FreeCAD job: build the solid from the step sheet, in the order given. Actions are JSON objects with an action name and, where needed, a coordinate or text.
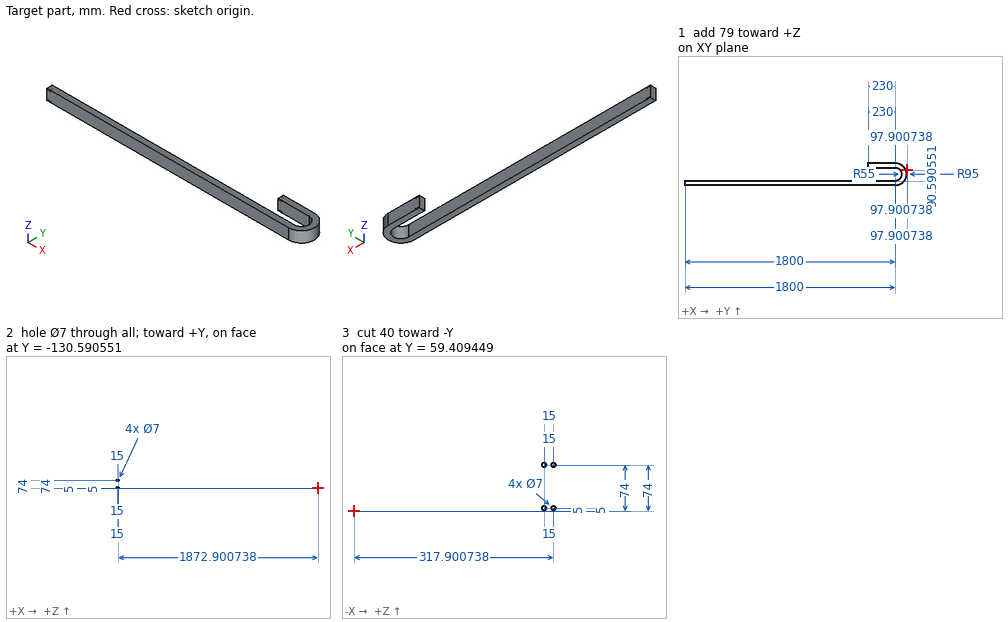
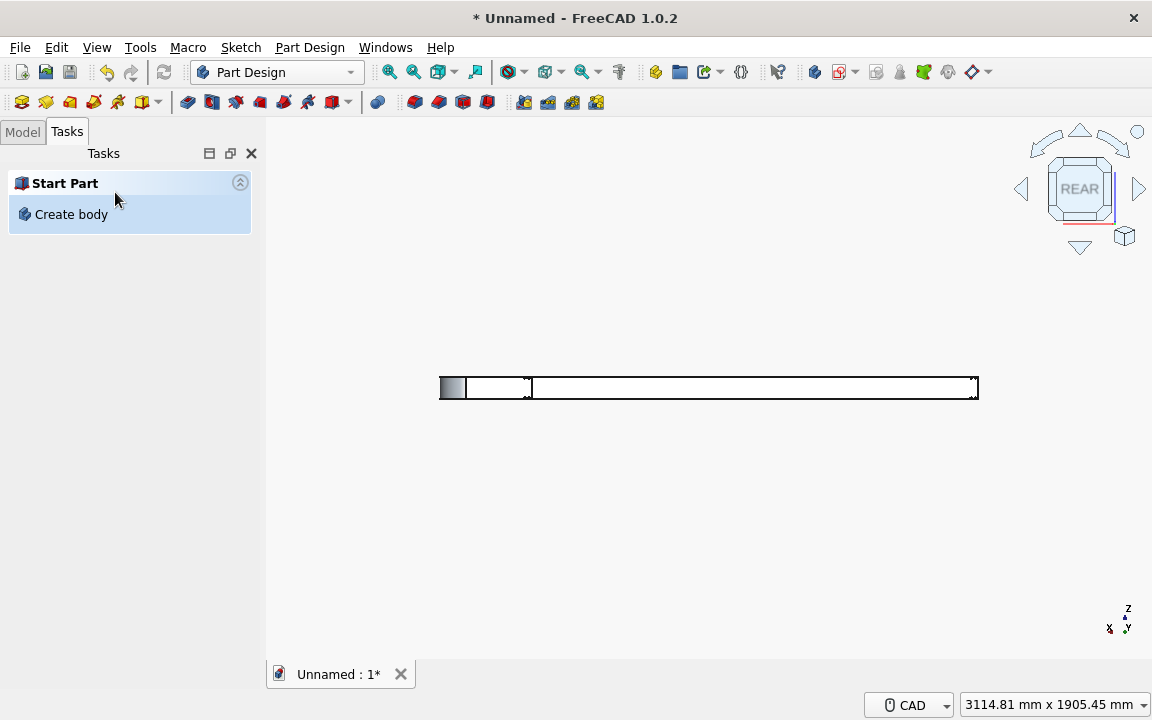
{"action": "key", "text": "0"}